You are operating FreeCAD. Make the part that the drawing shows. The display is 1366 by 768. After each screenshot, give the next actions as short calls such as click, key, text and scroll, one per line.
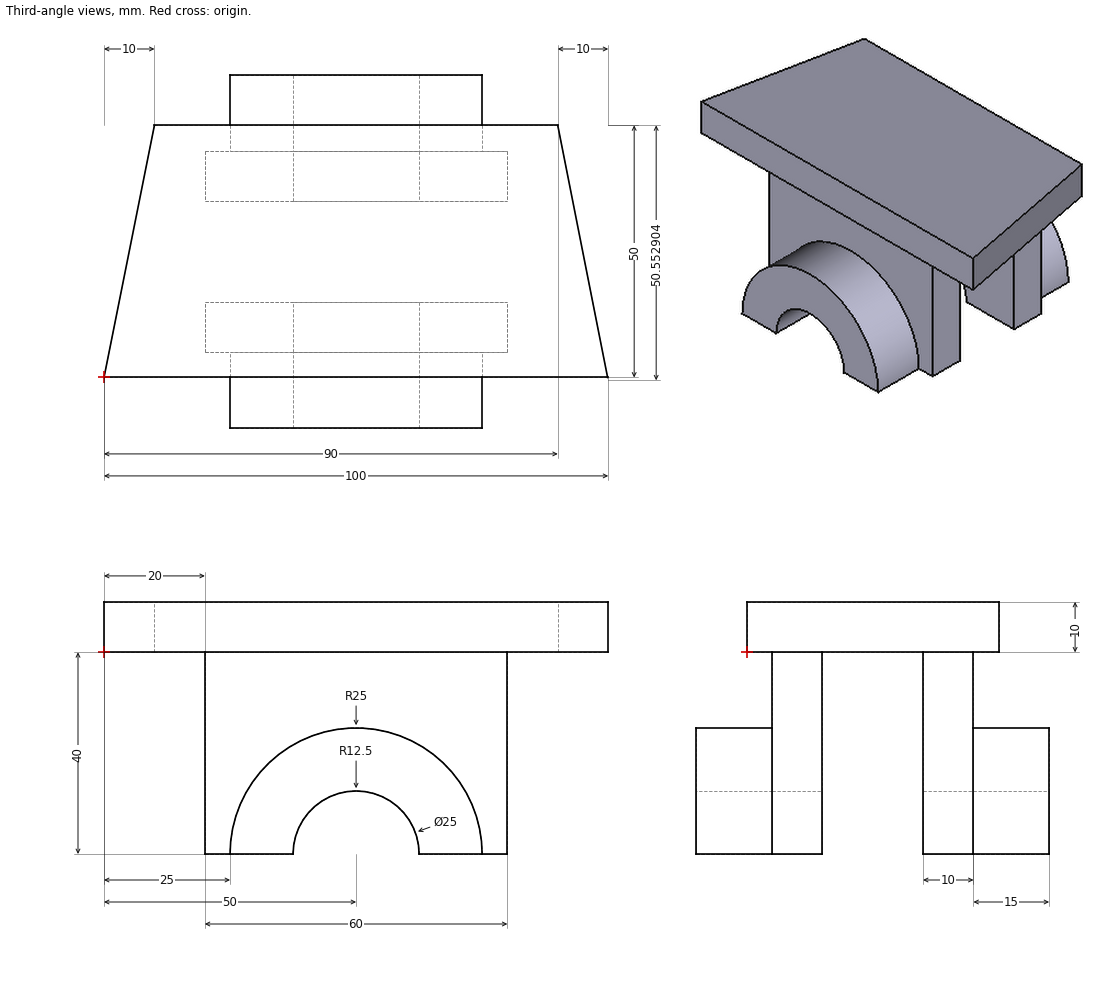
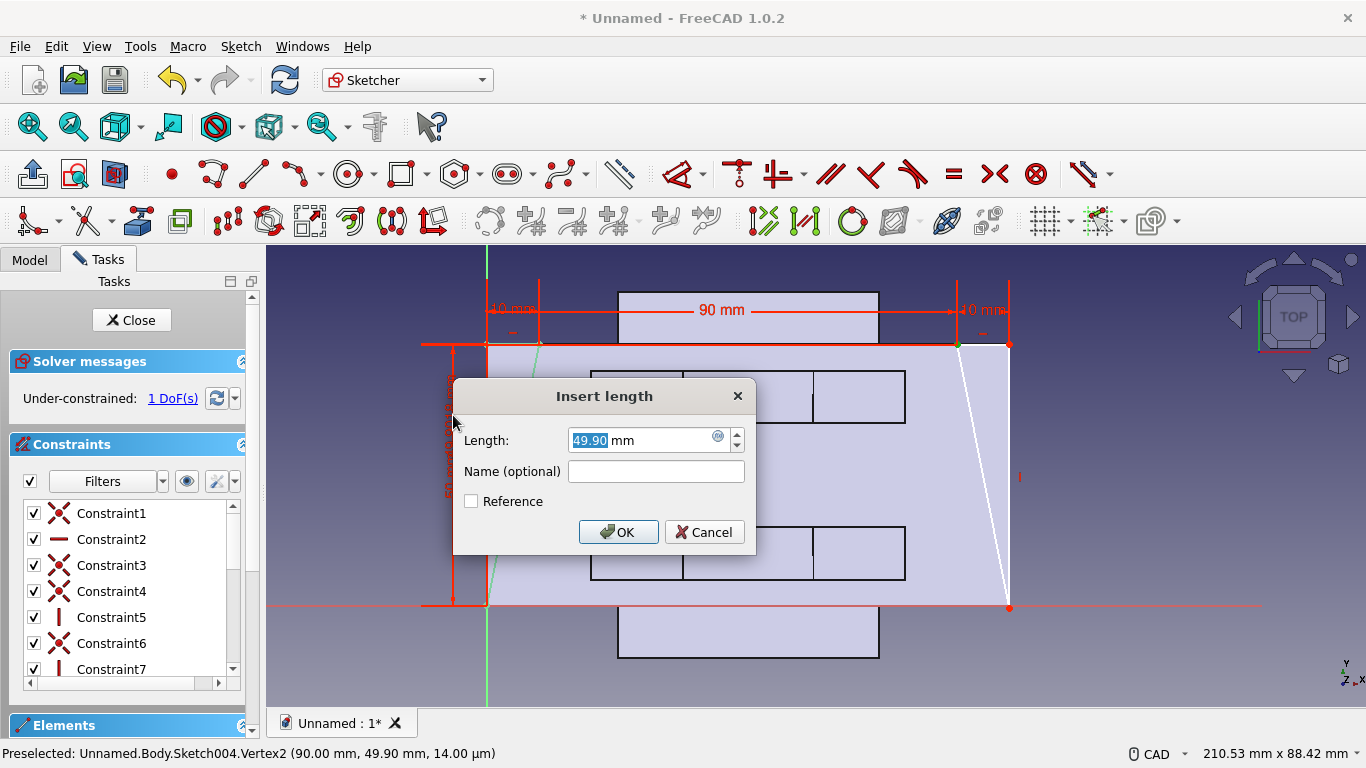
text(50)
key(Return)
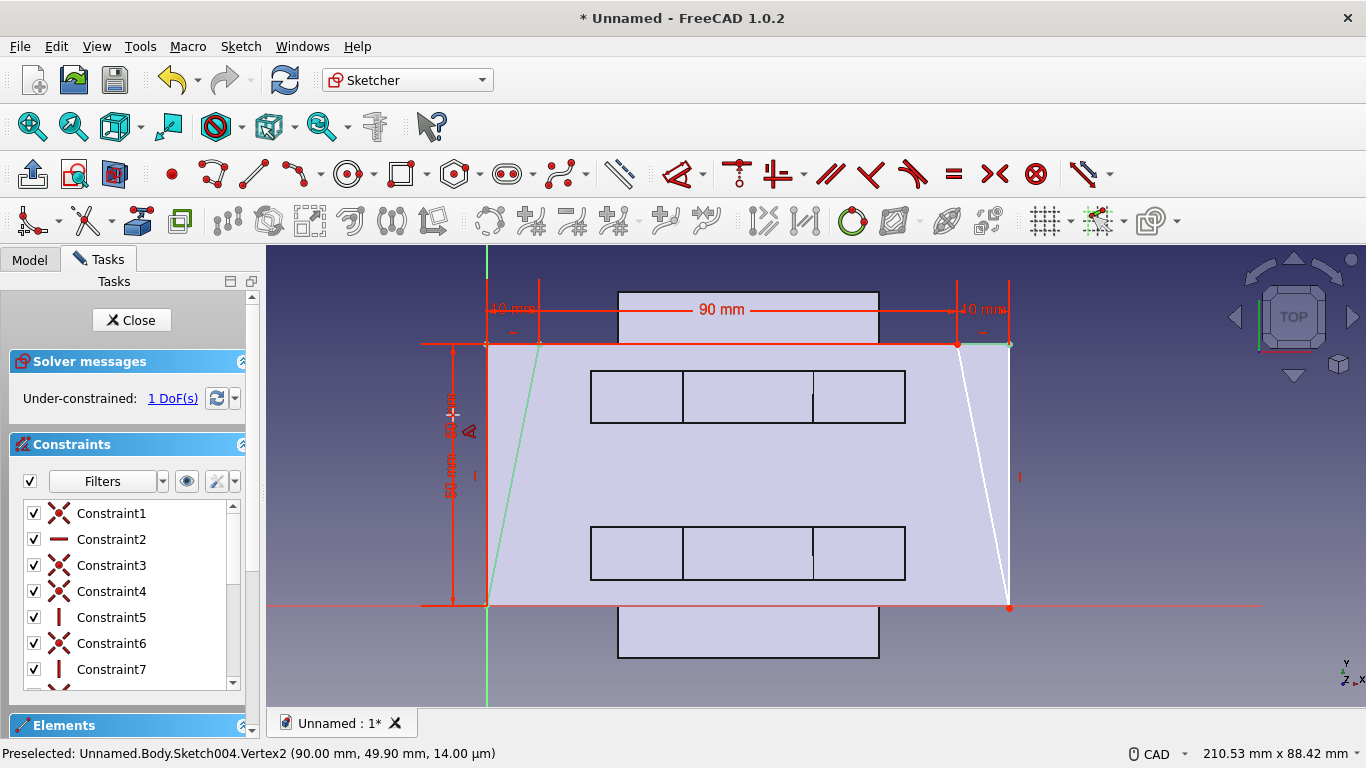
click(1009, 424)
click(1043, 477)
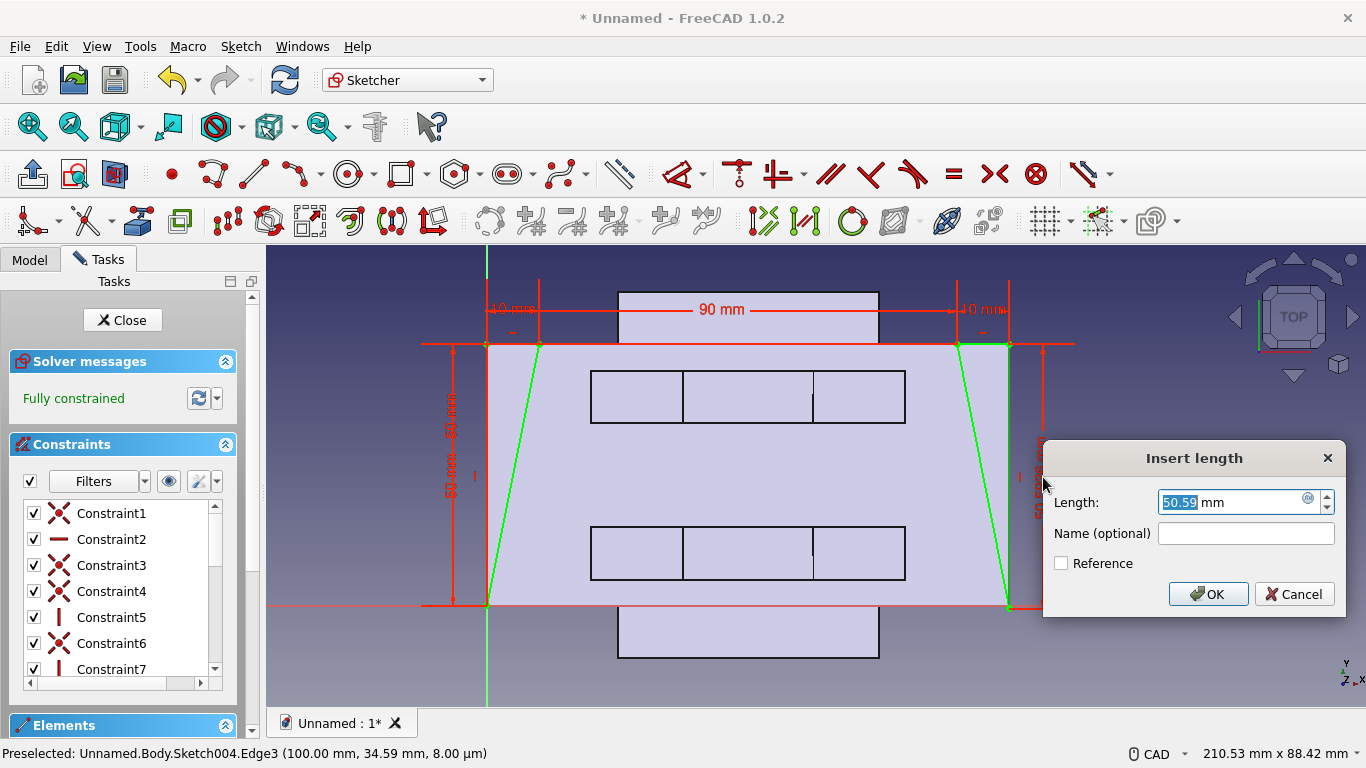
text(50.552904)
key(Return)
key(Escape)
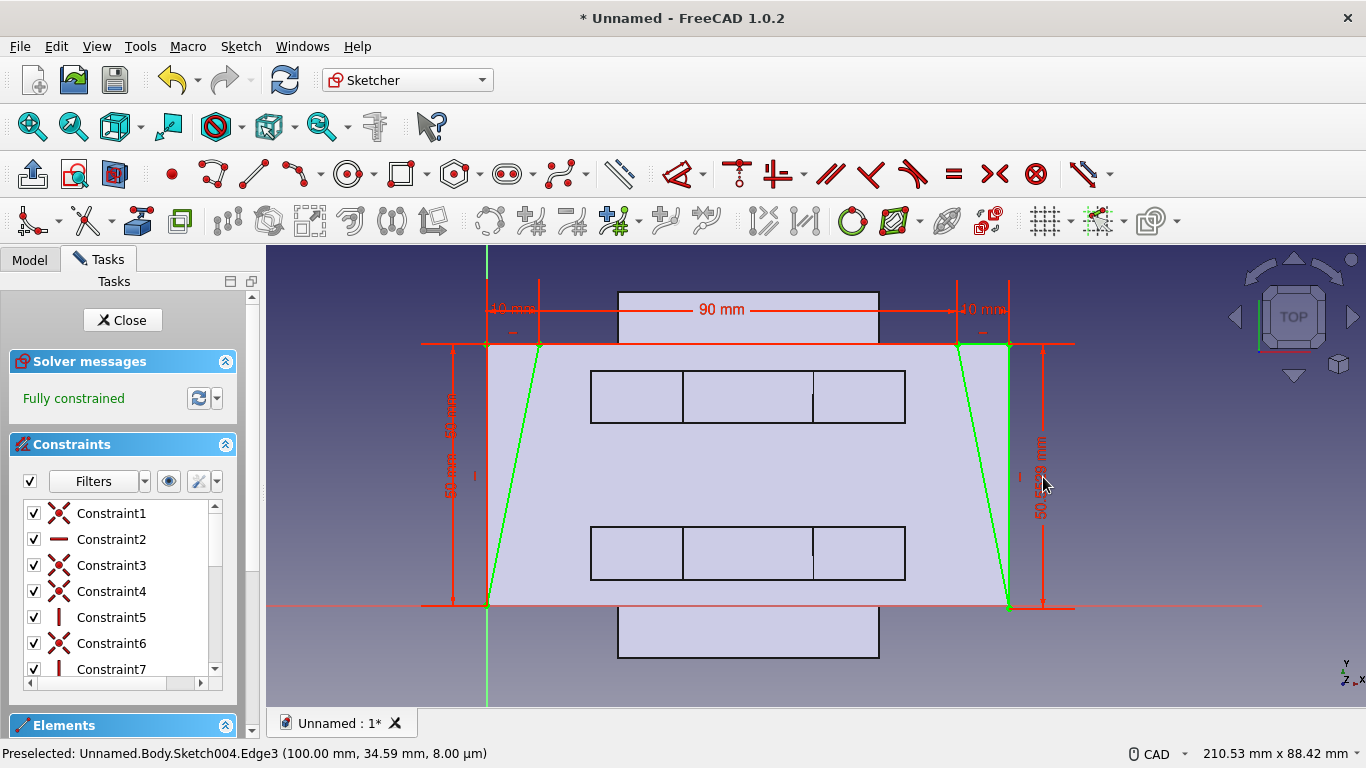
click(123, 320)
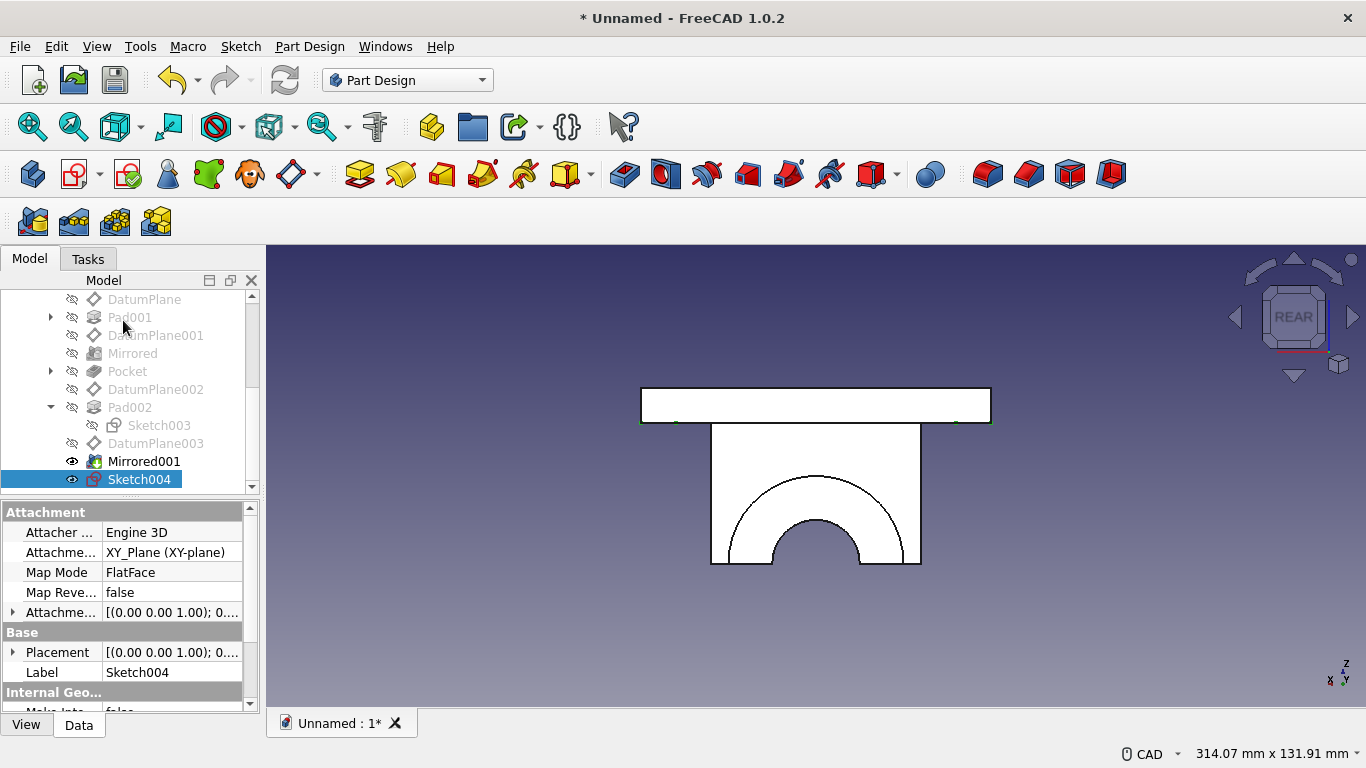
click(625, 174)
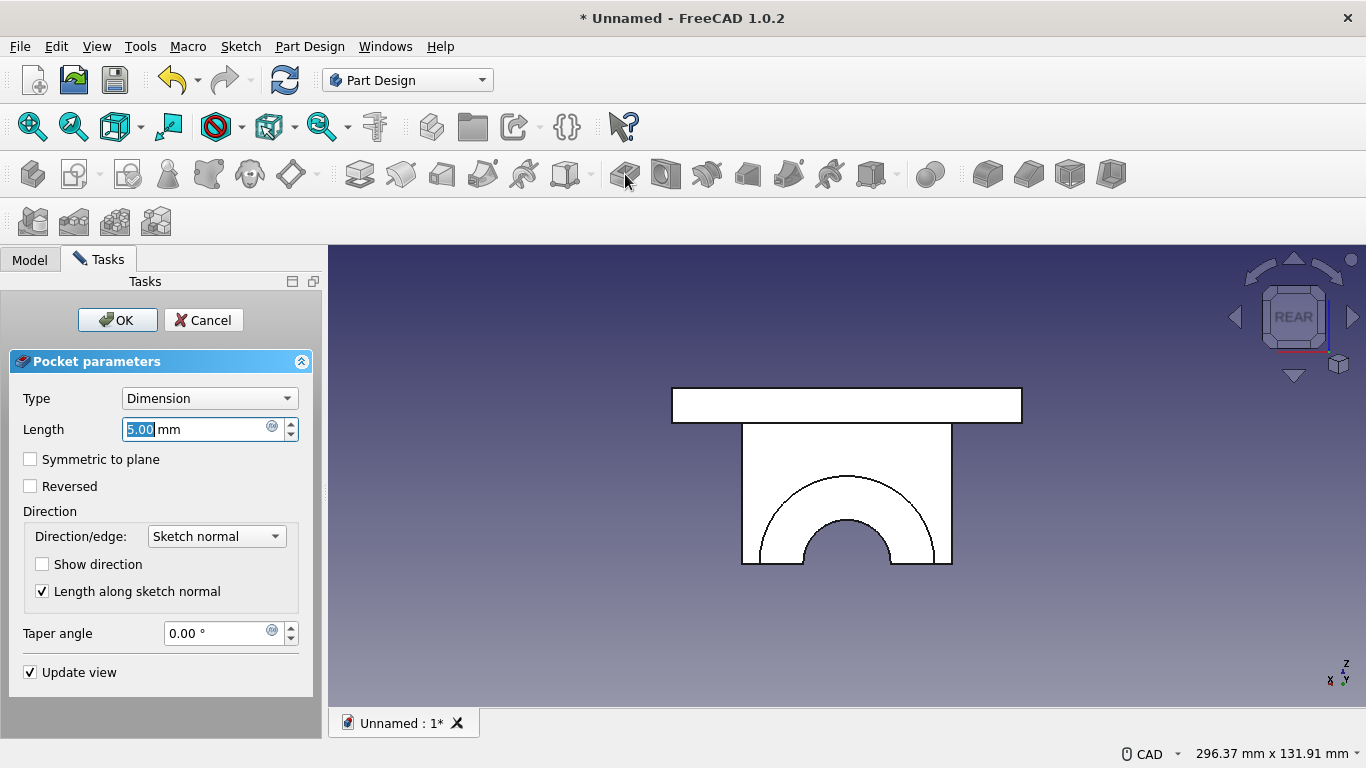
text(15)
key(Tab)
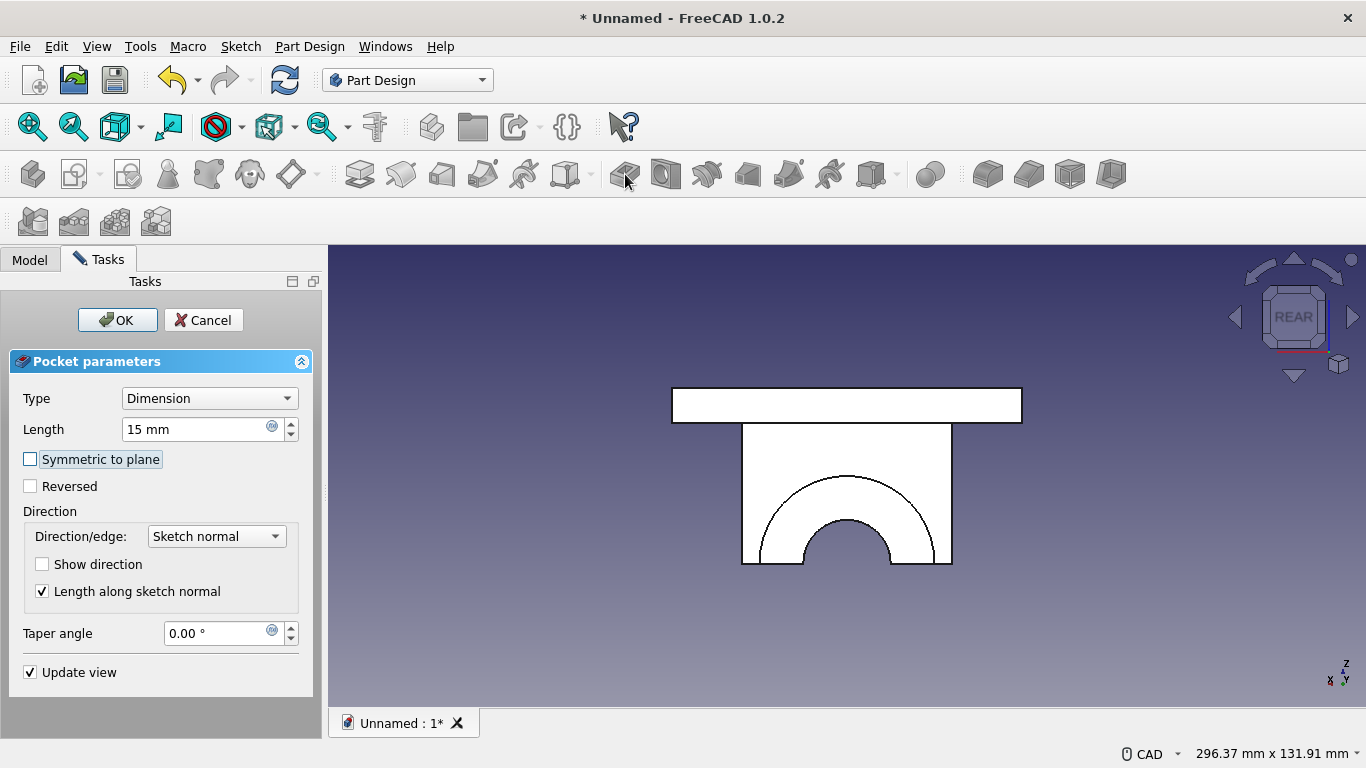
click(31, 486)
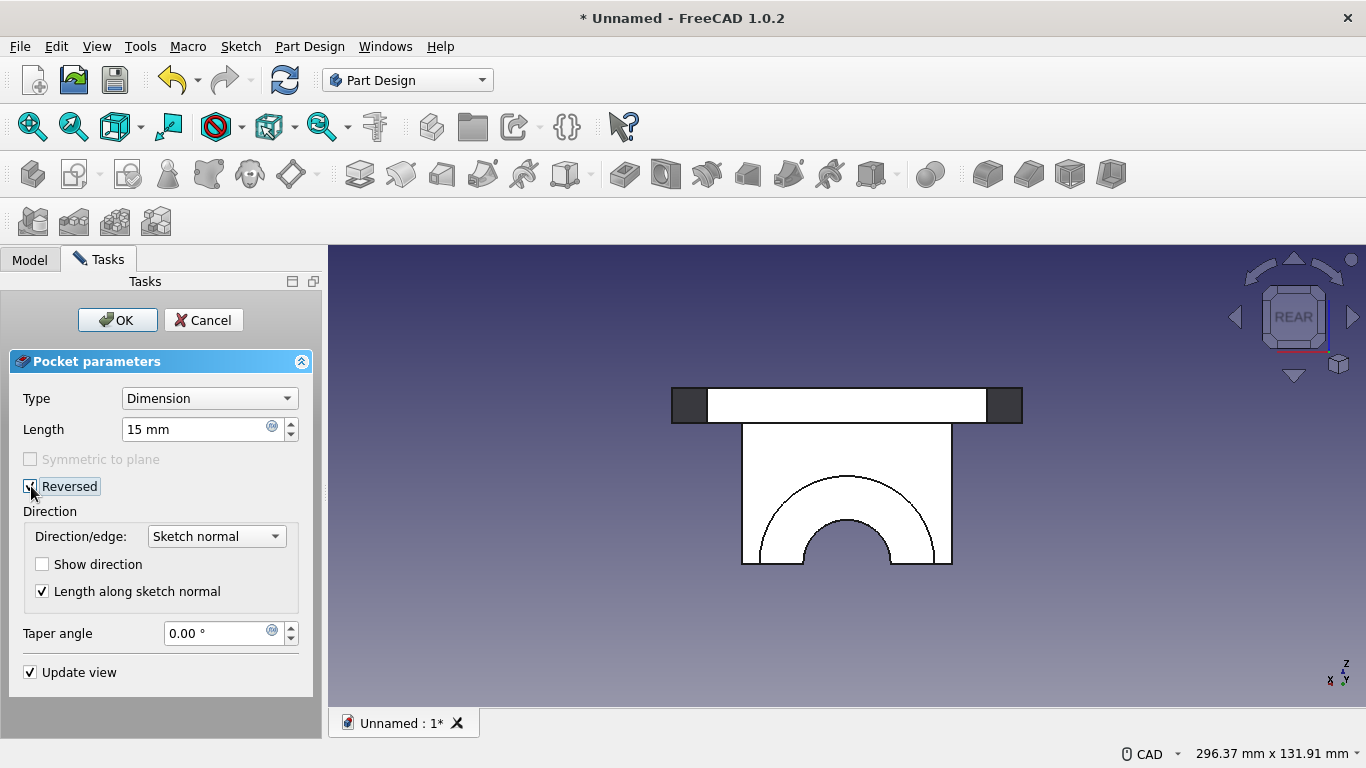
click(118, 320)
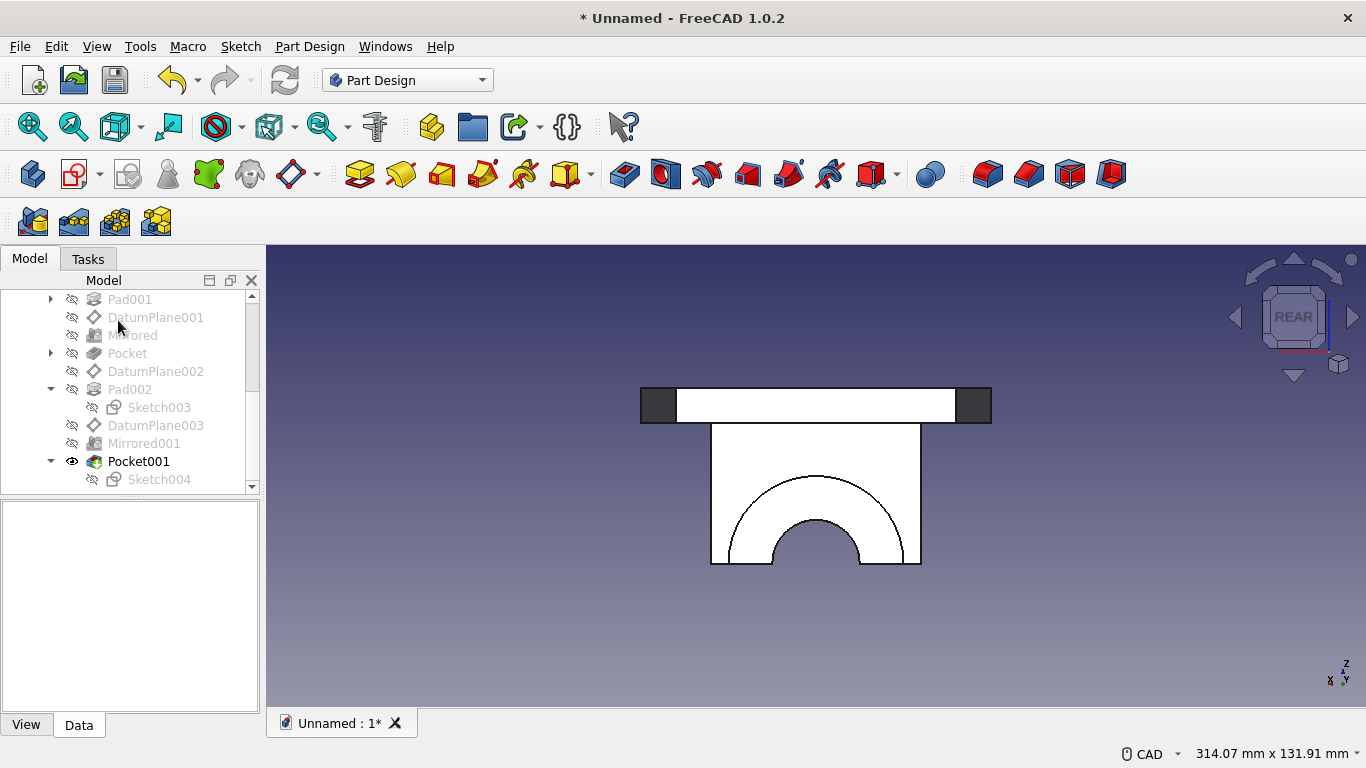
key(0)